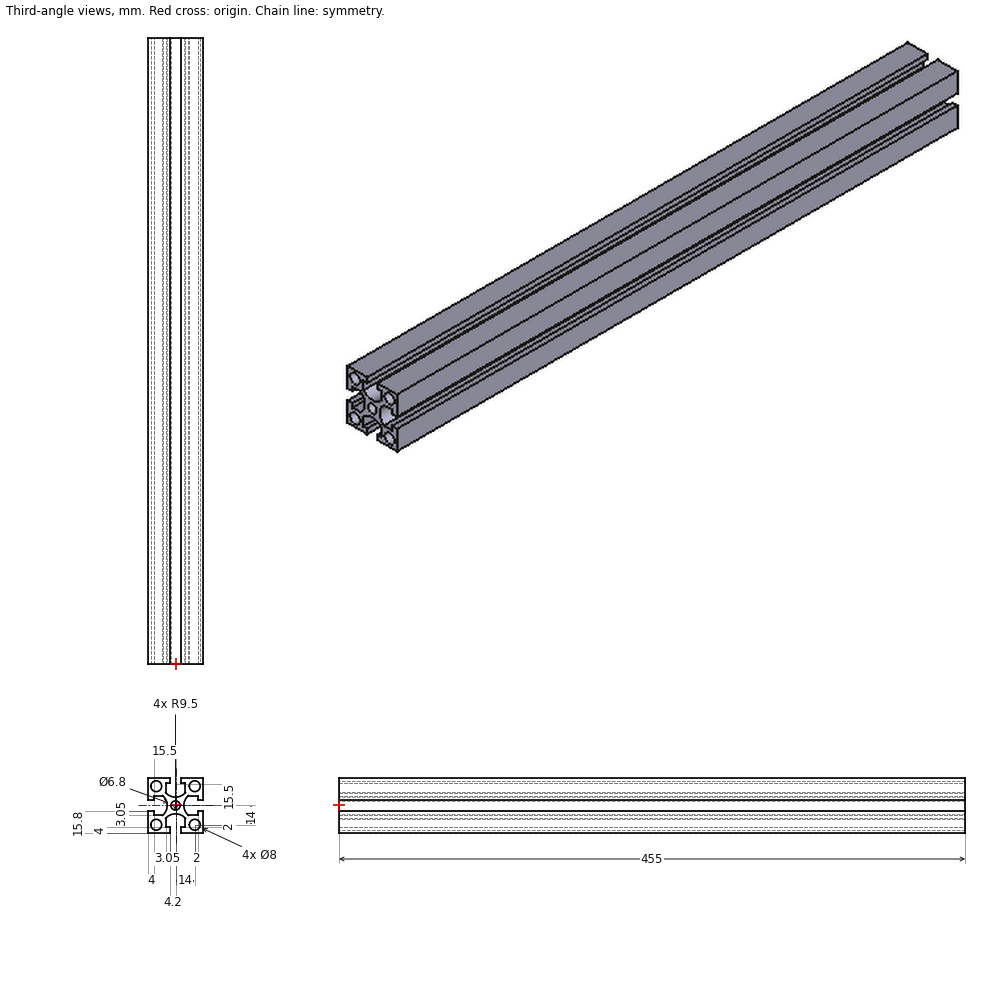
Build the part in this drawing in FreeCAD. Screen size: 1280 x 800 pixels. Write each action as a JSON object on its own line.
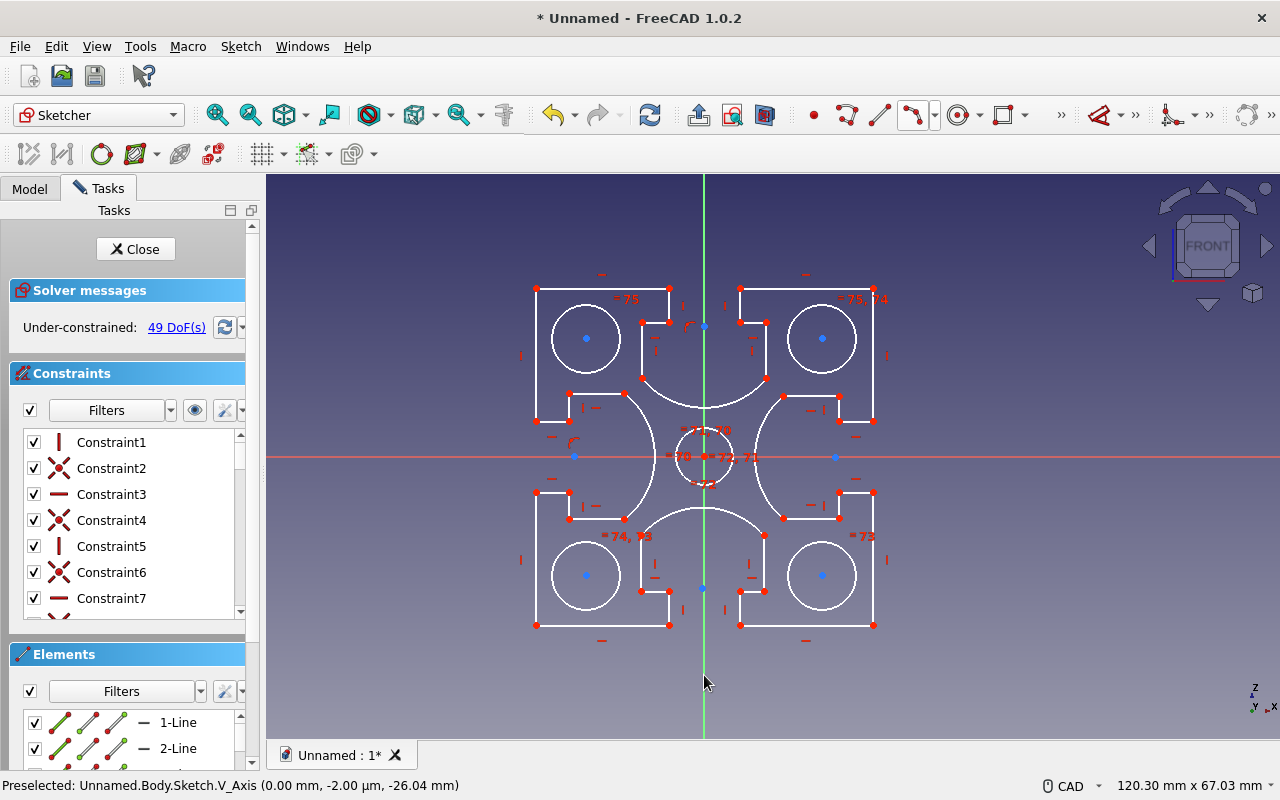
{"action": "left_click", "coordinate": [836, 458]}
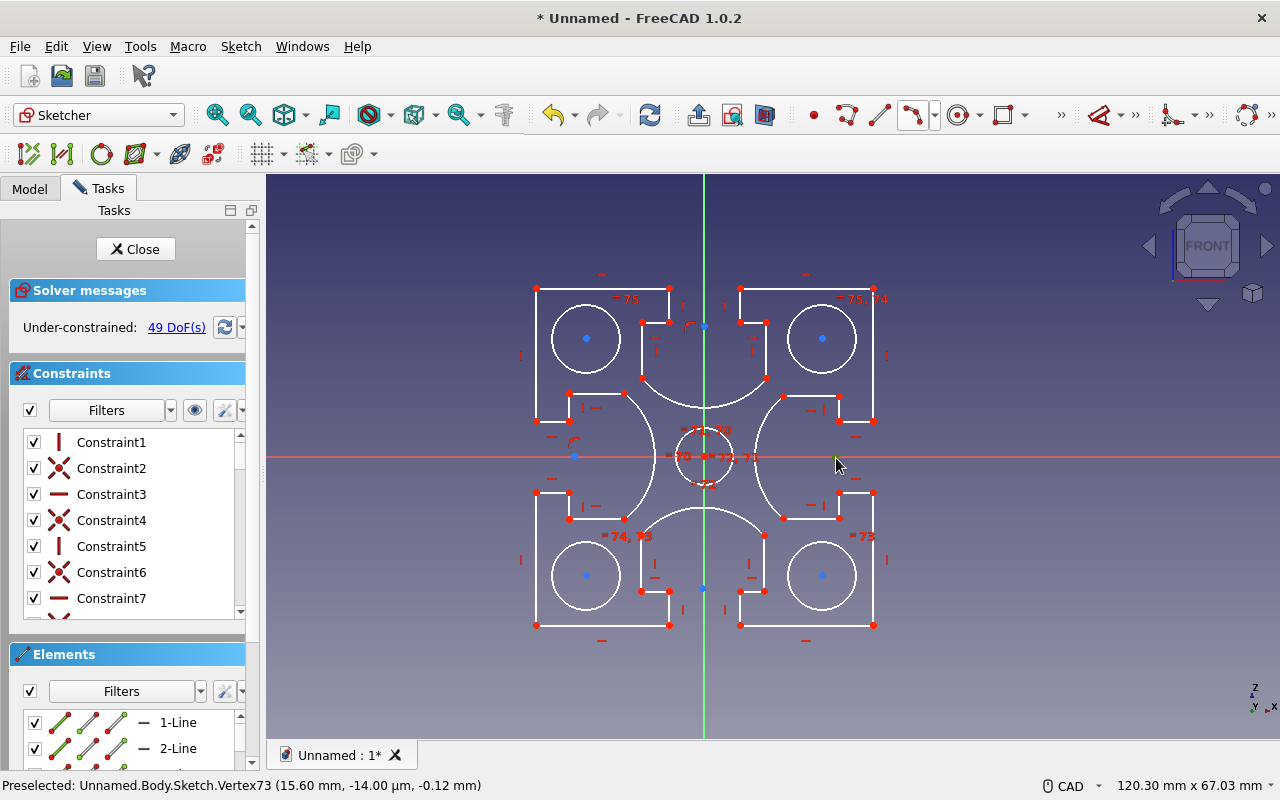
{"action": "left_click", "coordinate": [353, 456]}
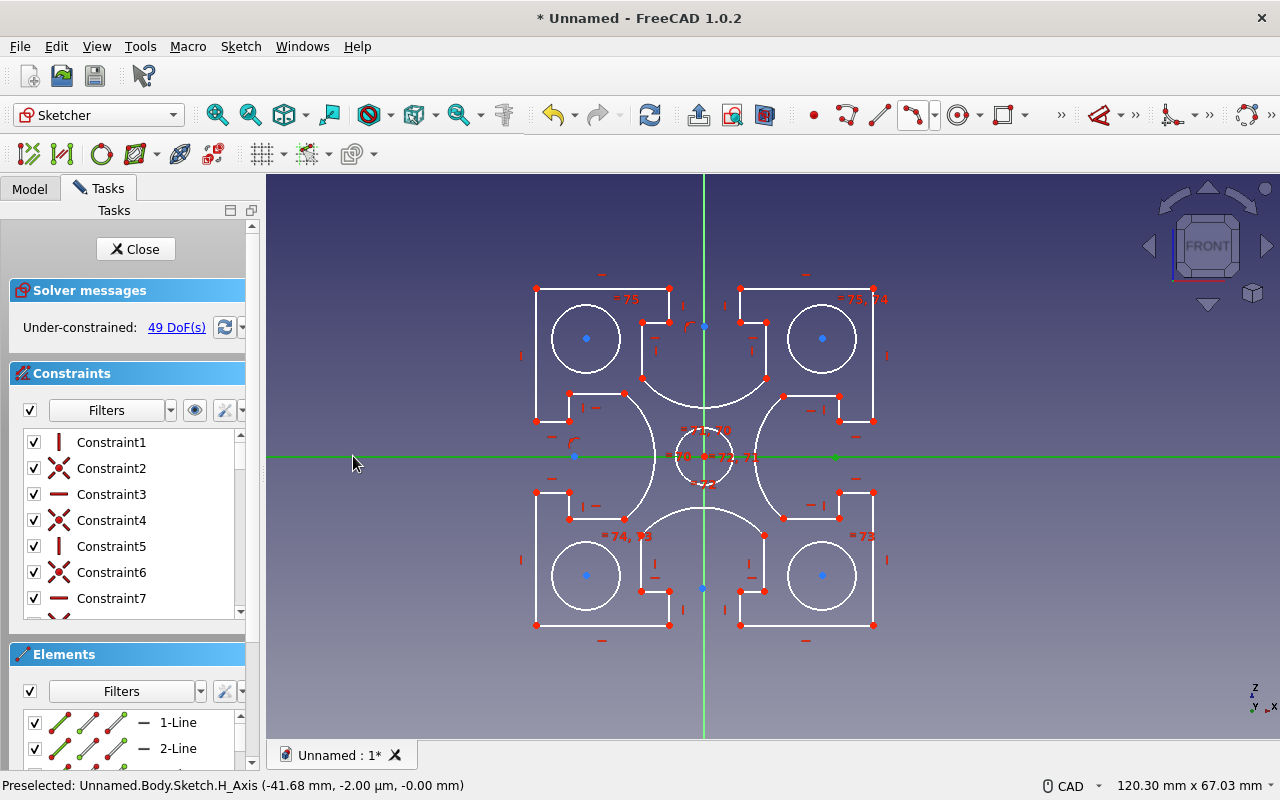
{"action": "key", "text": "c"}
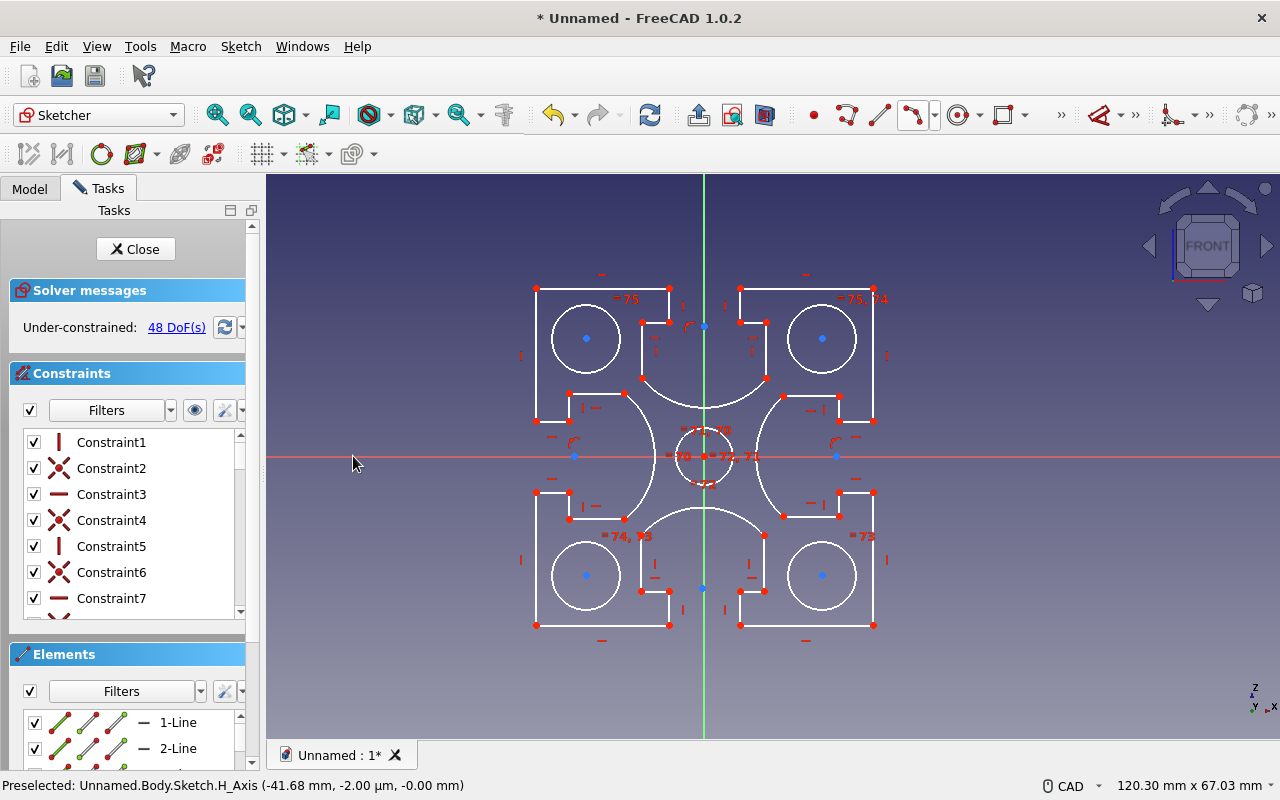
{"action": "left_click", "coordinate": [703, 588]}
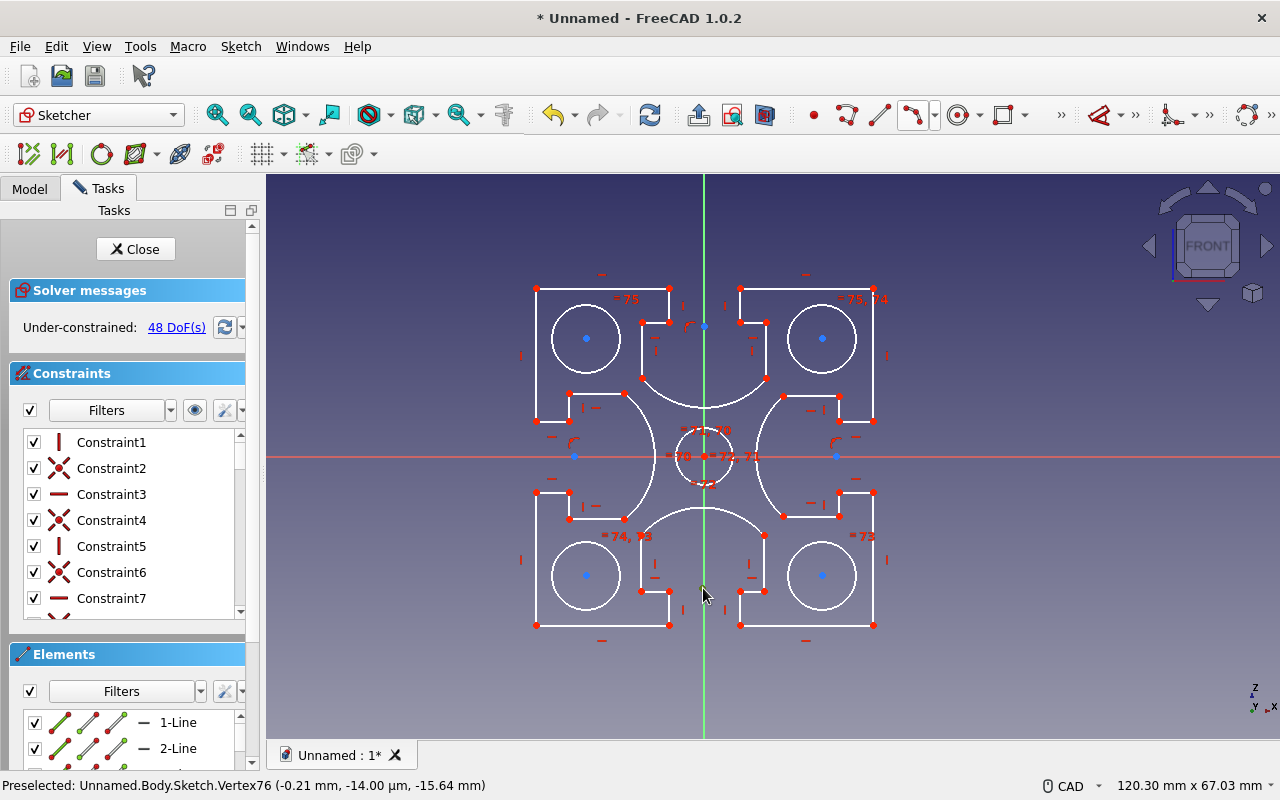
{"action": "left_click", "coordinate": [704, 675]}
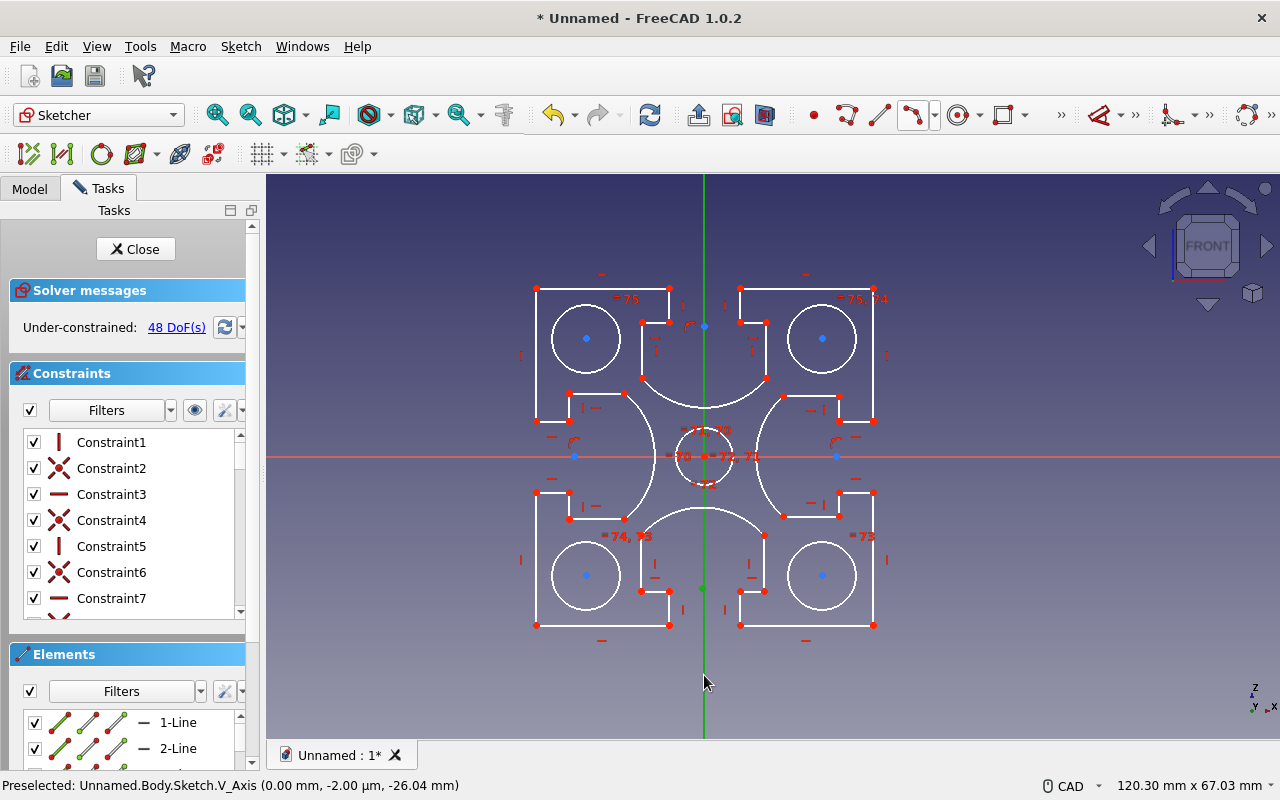
{"action": "key", "text": "c"}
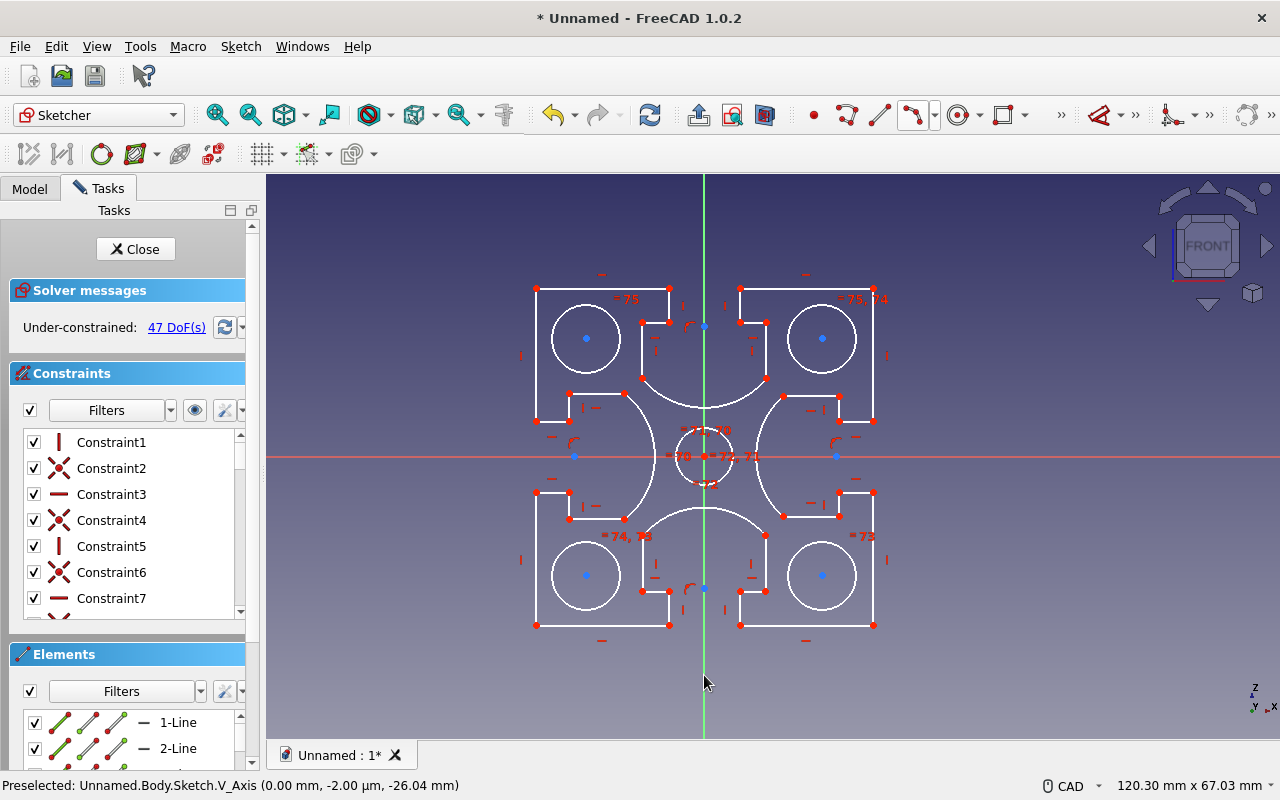
{"action": "left_click", "coordinate": [822, 576]}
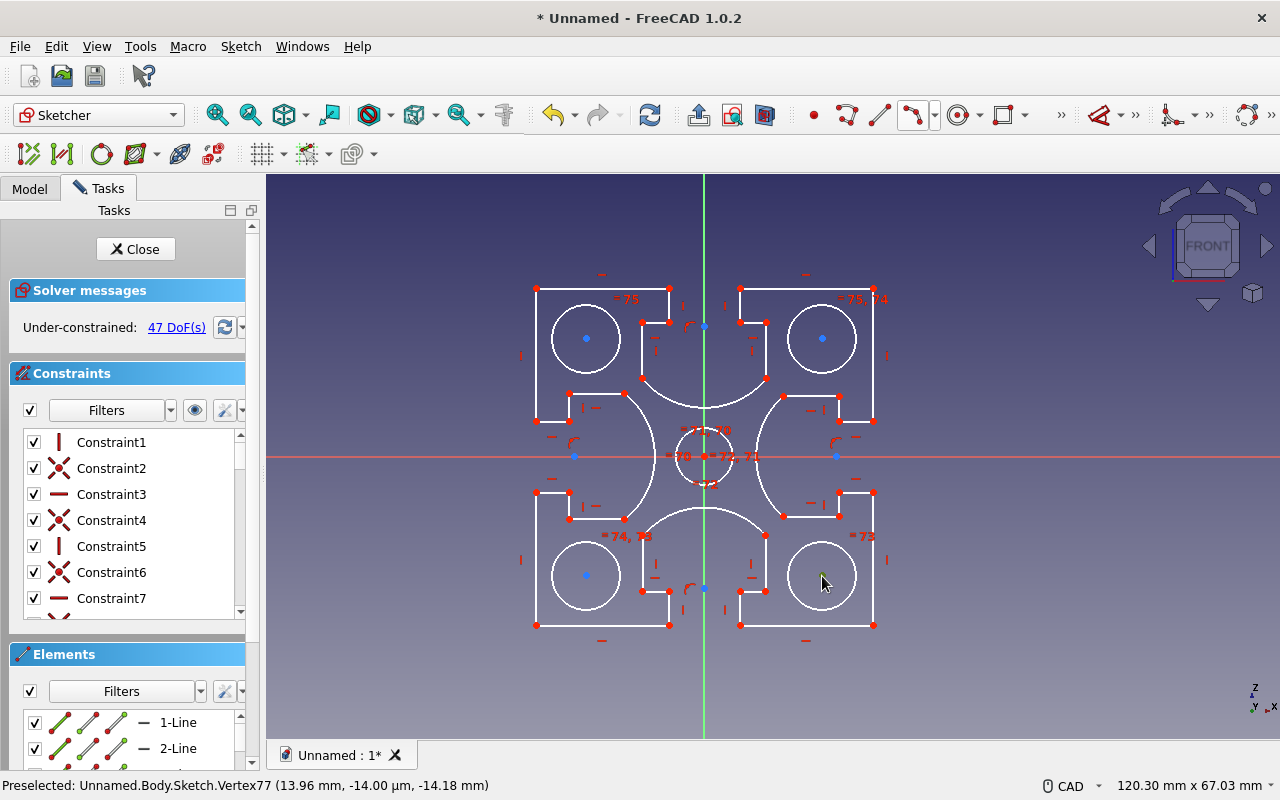
{"action": "left_click", "coordinate": [586, 576]}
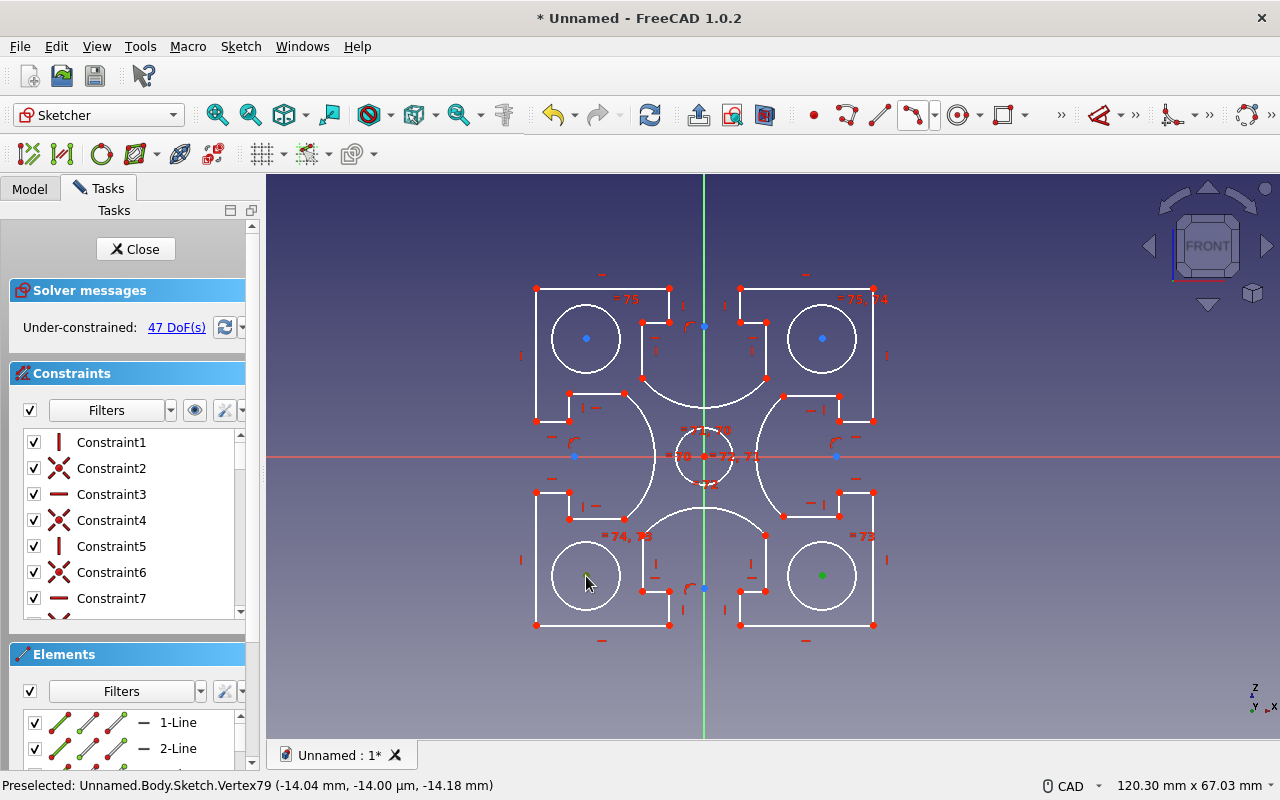
{"action": "left_click", "coordinate": [704, 675]}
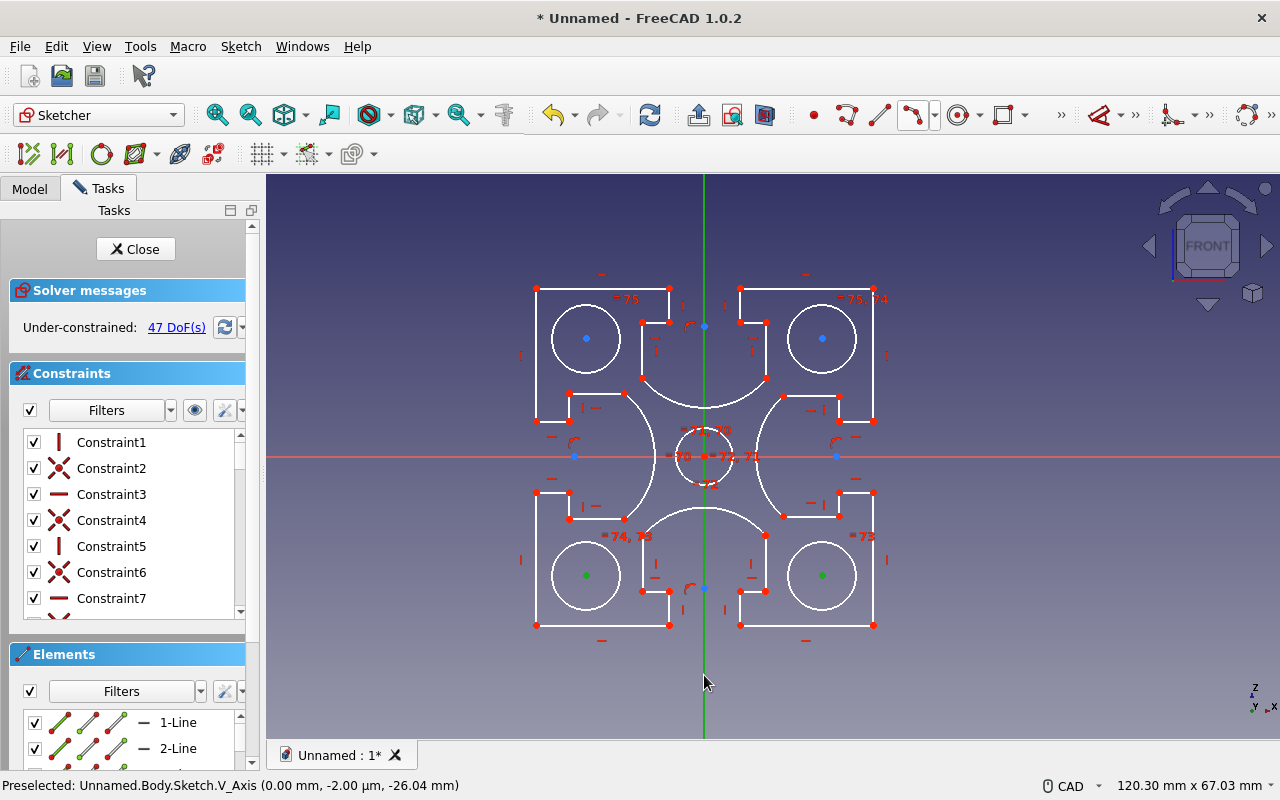
{"action": "key", "text": "s"}